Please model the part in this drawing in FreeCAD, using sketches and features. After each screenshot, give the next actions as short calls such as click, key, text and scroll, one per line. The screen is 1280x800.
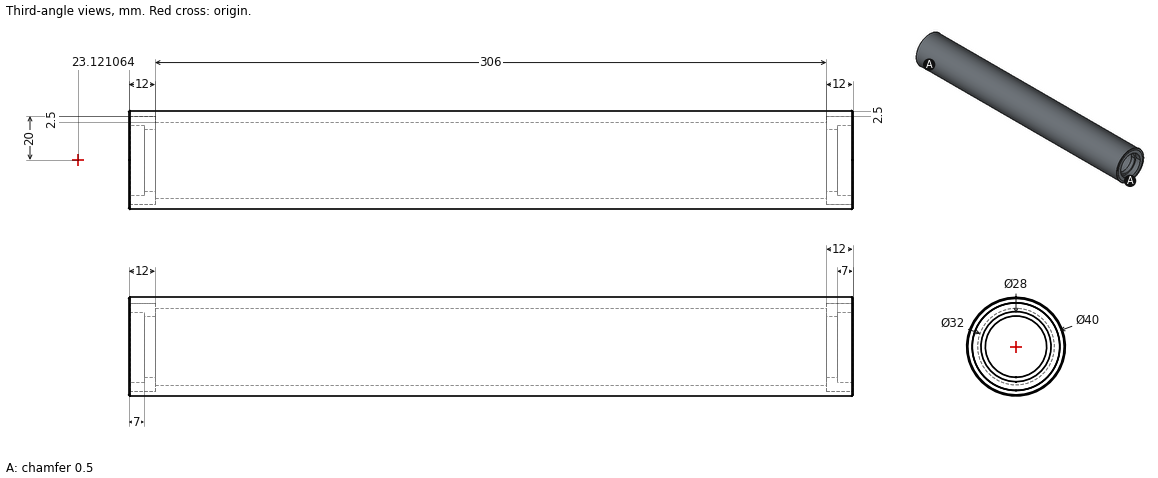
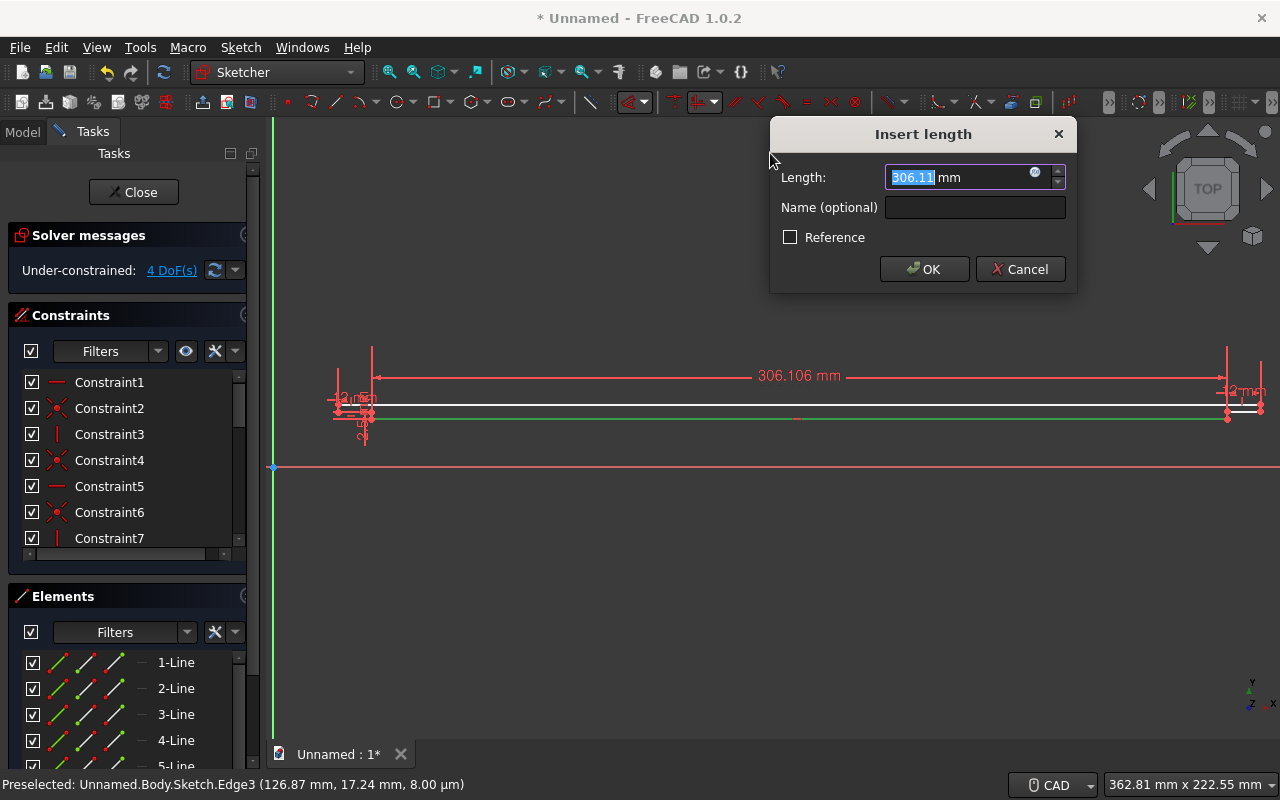
text(306)
key(Return)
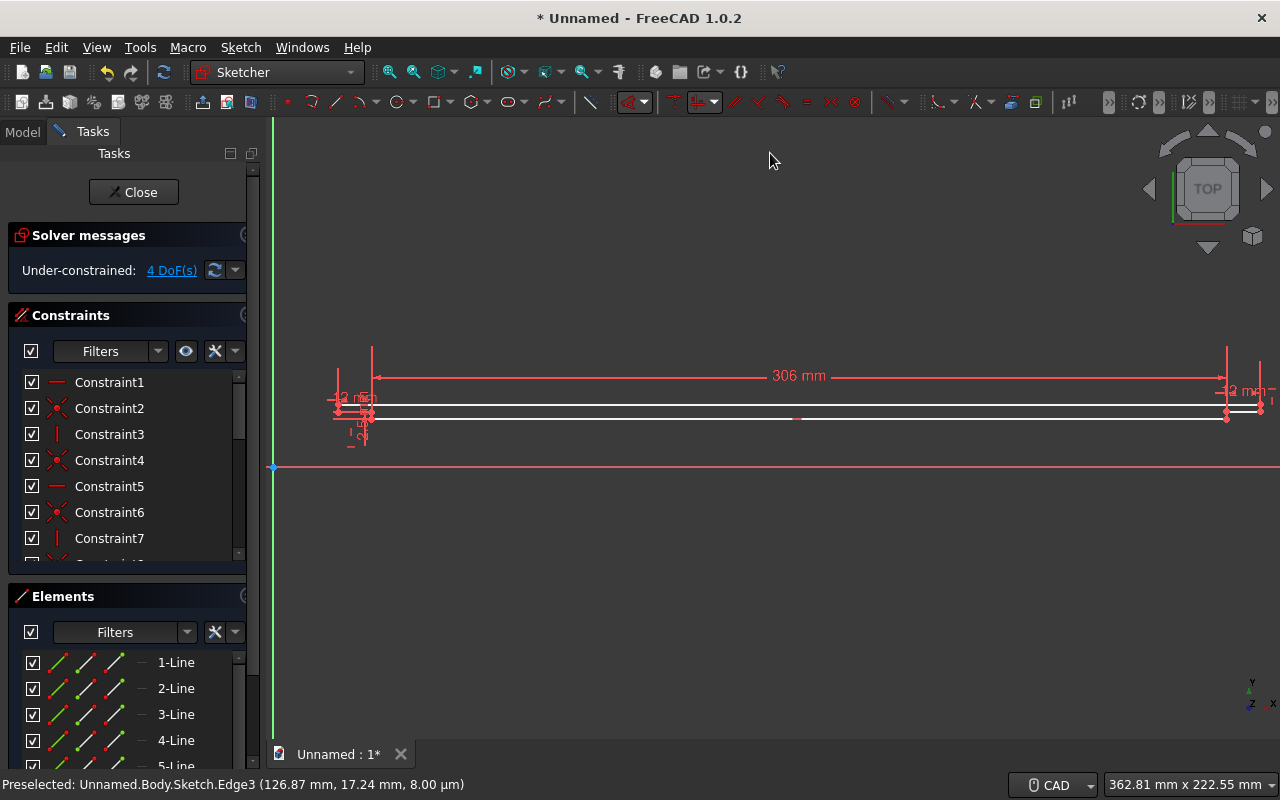
scroll(629, 418, down, 3)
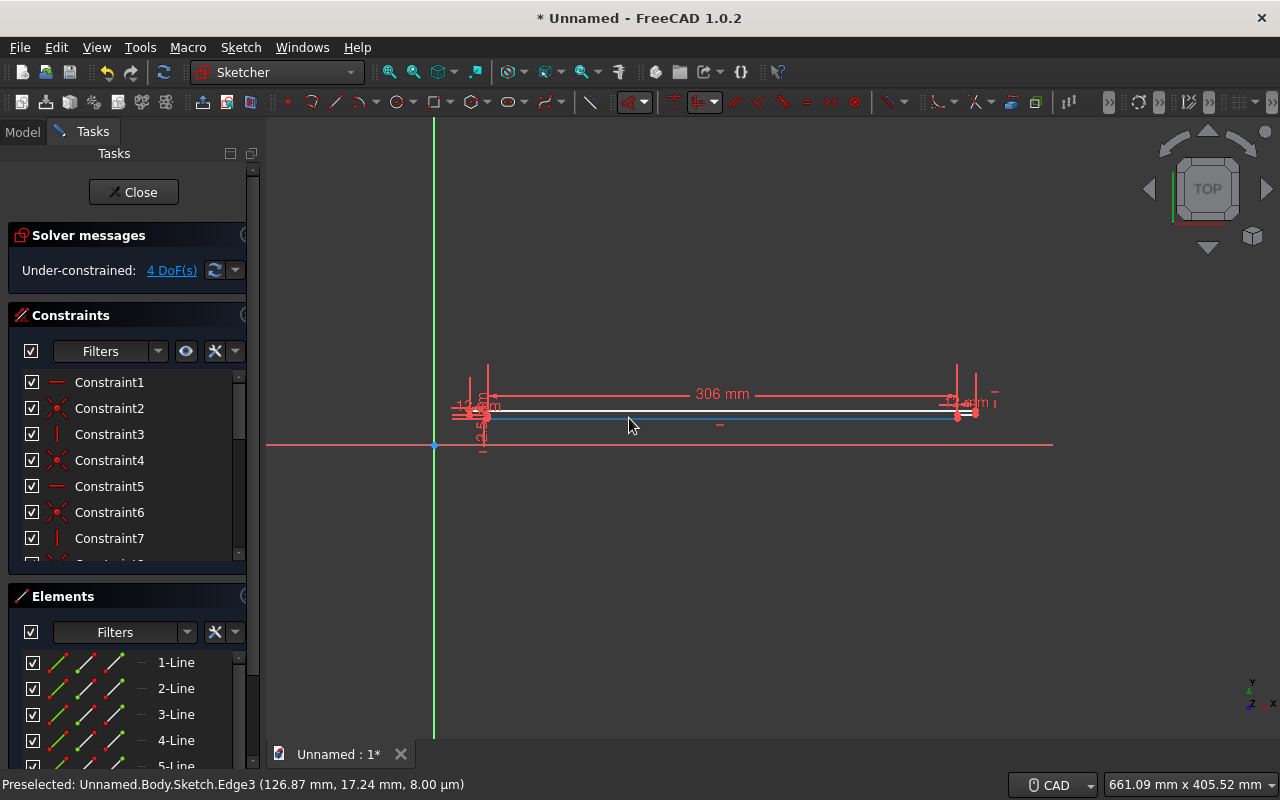
scroll(957, 417, up, 12)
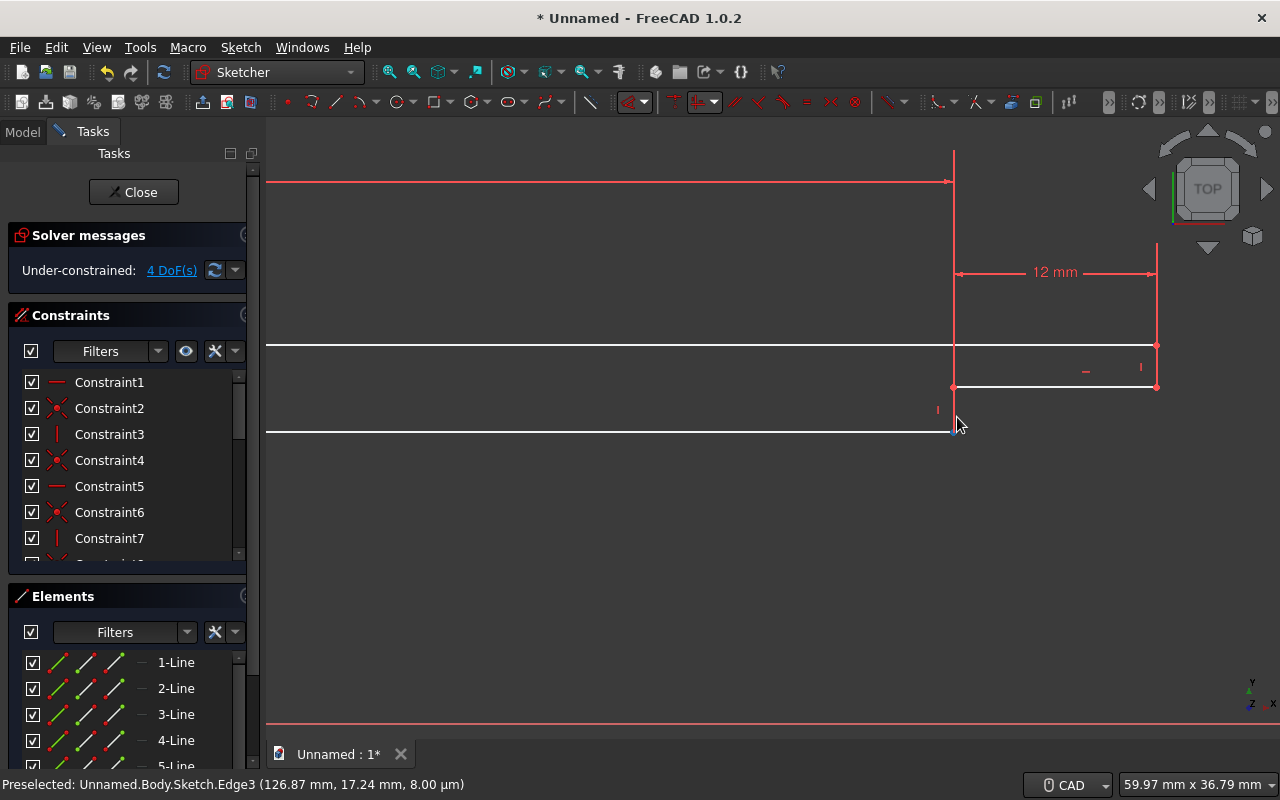
click(954, 410)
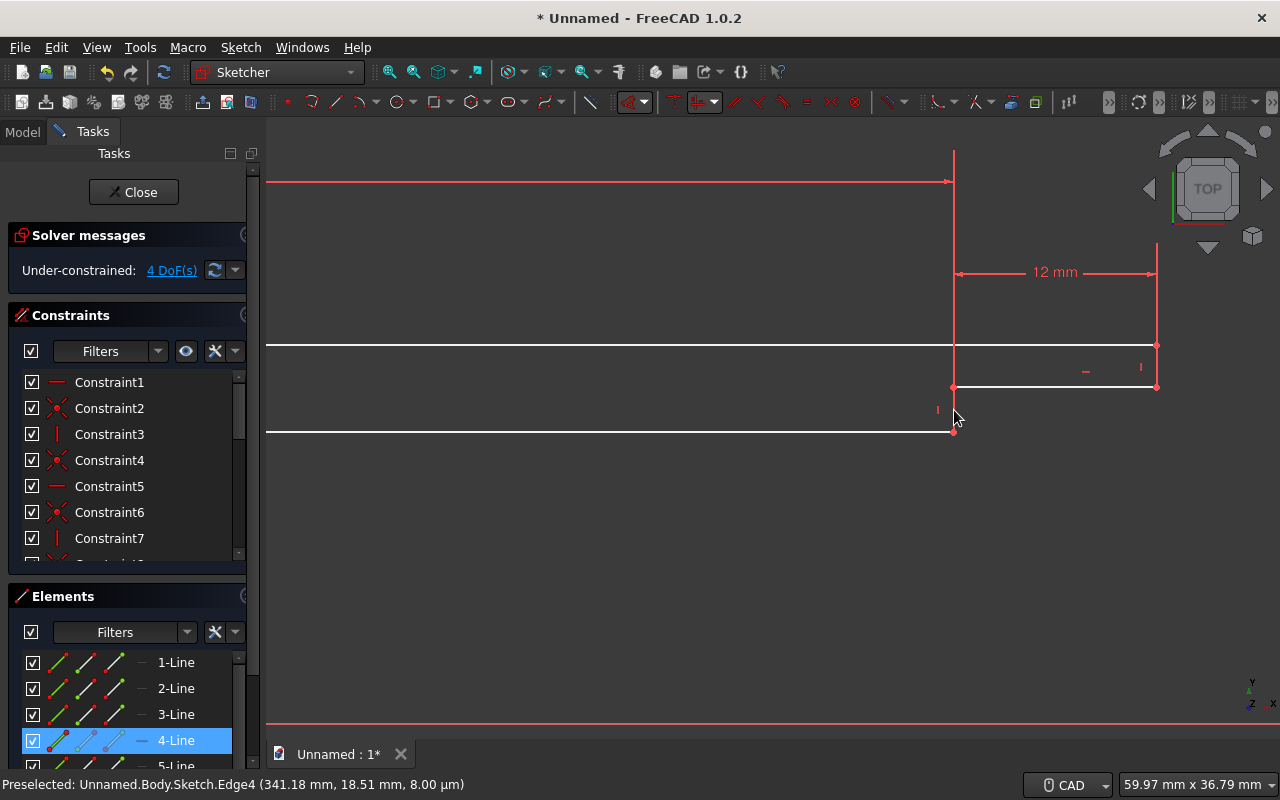
click(646, 102)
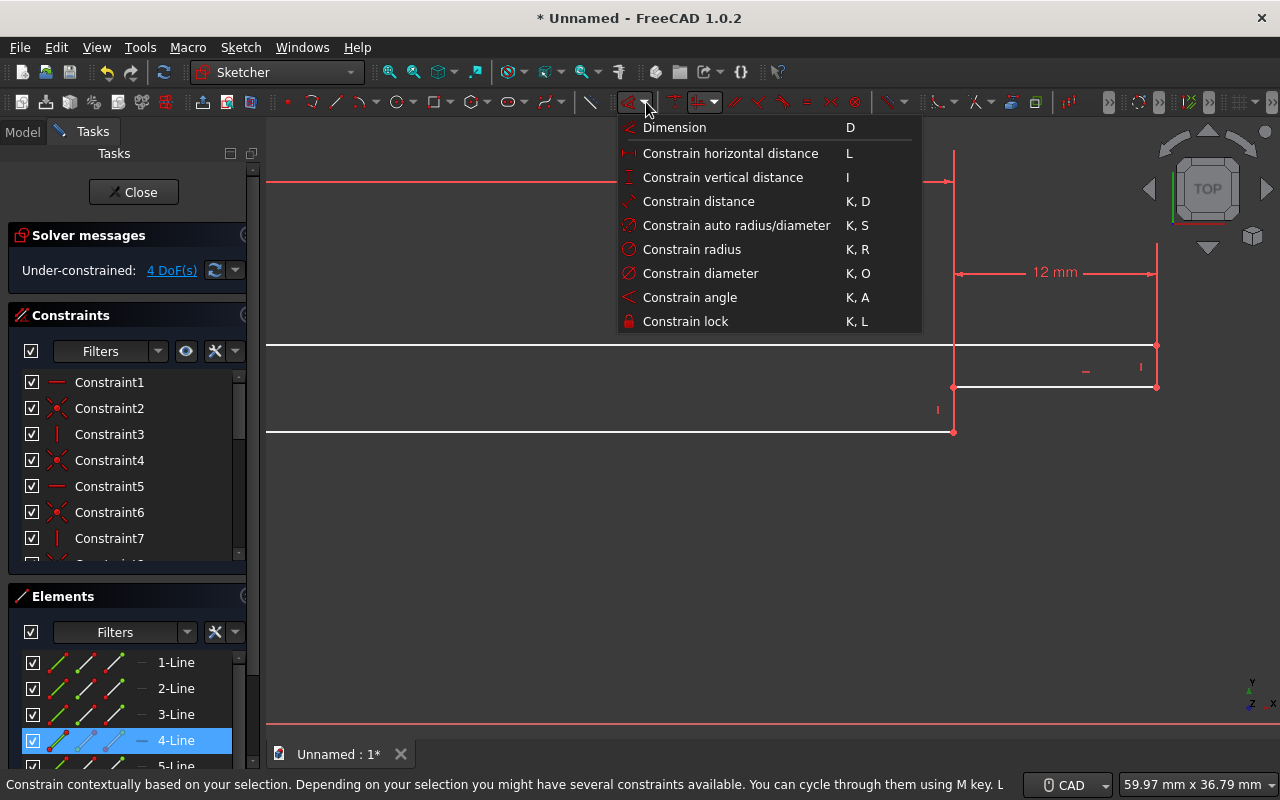
click(770, 177)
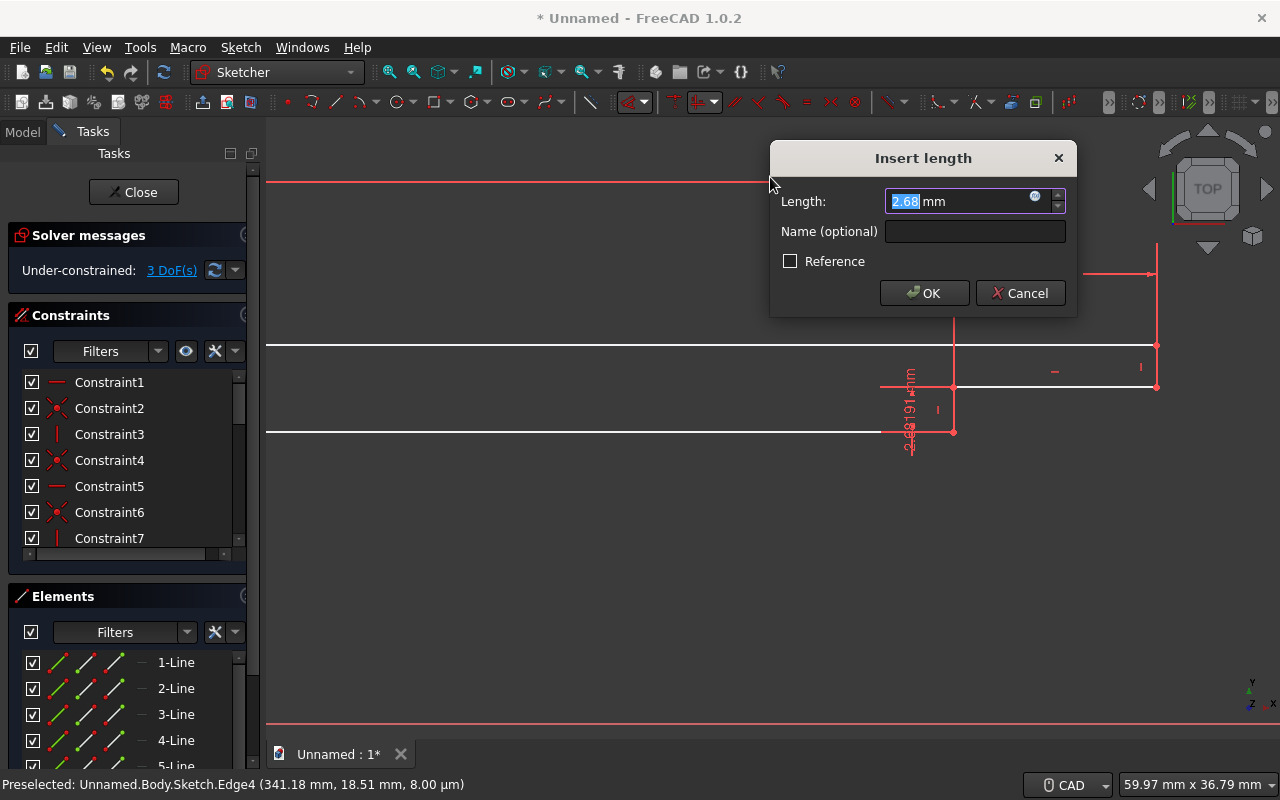
text(2.5)
key(Return)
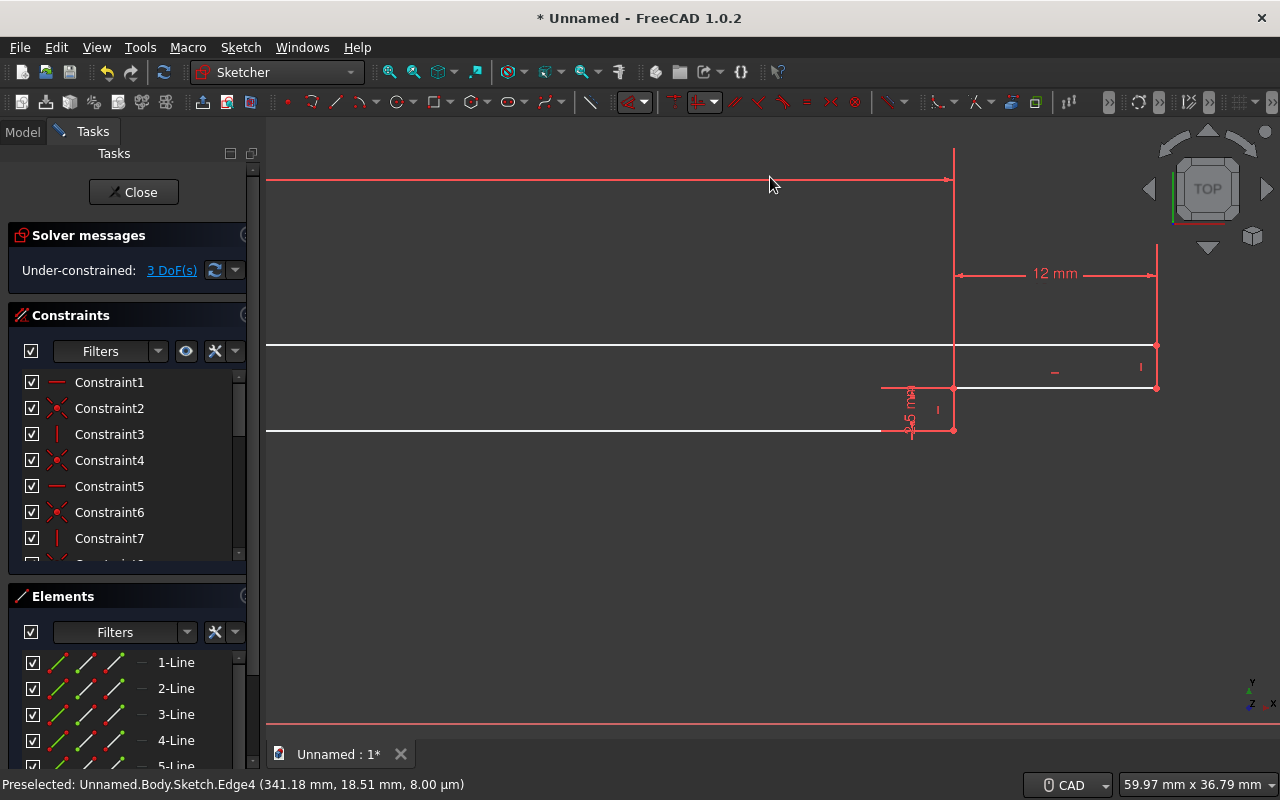
scroll(957, 417, down, 12)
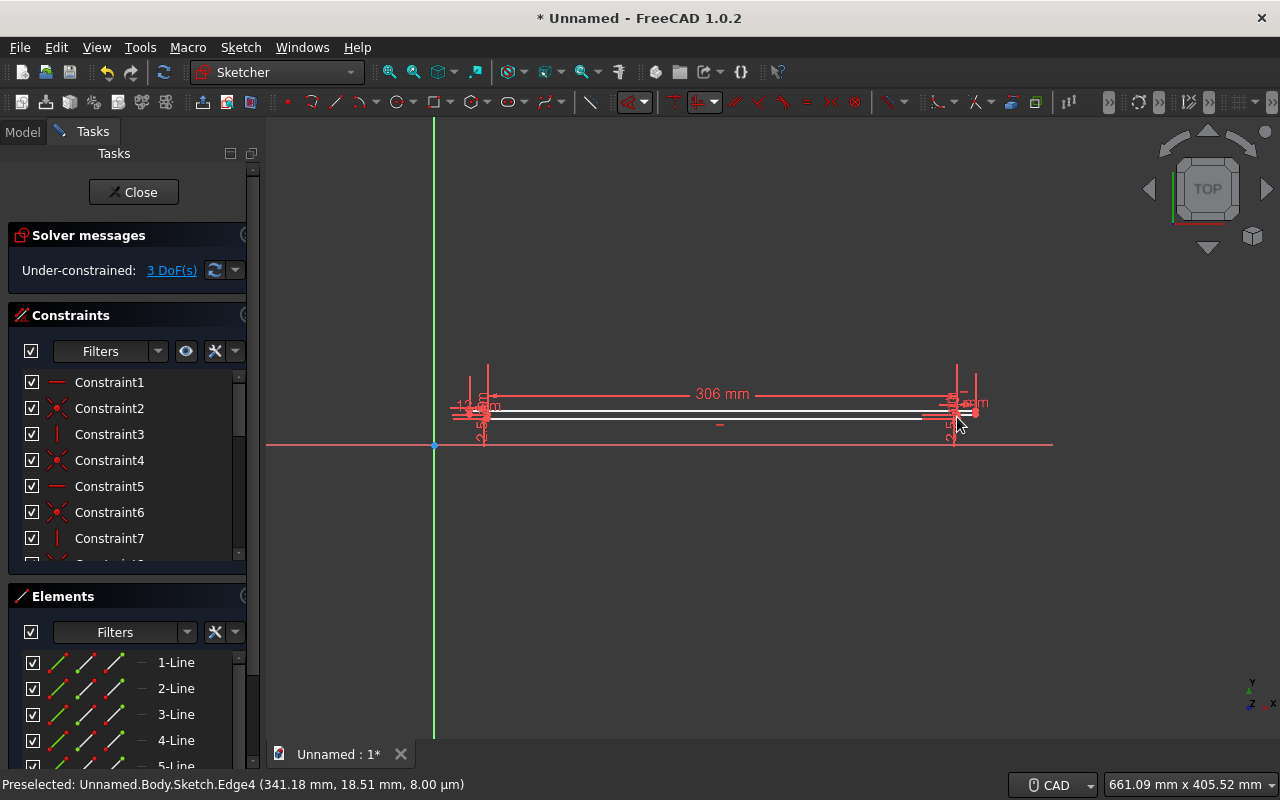
scroll(976, 414, up, 13)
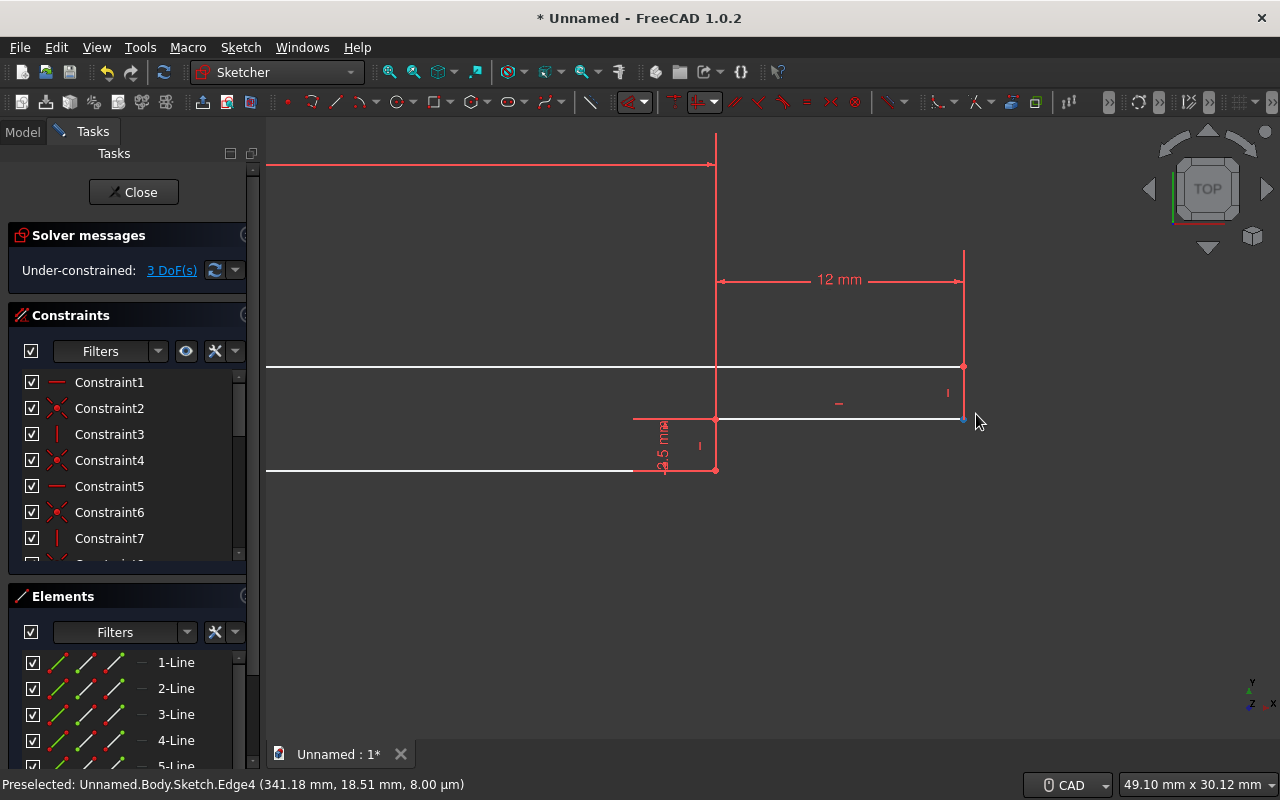
click(964, 404)